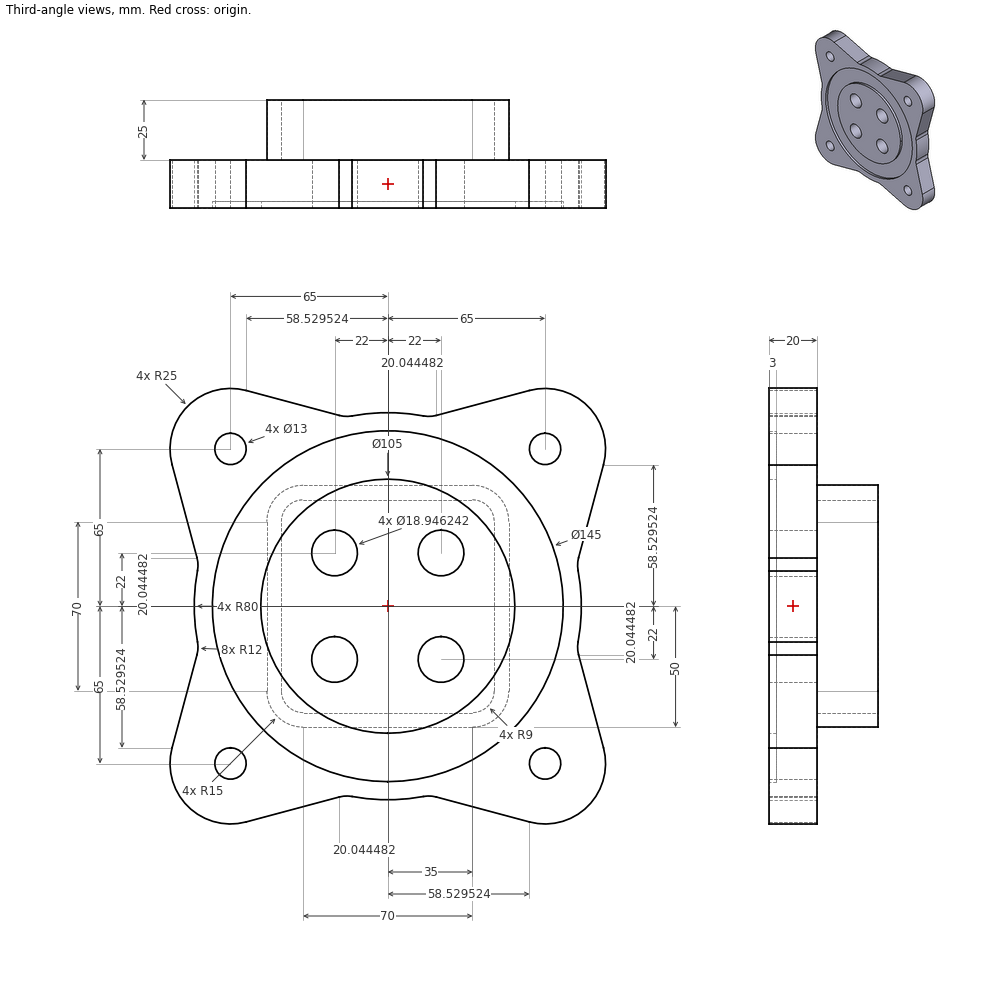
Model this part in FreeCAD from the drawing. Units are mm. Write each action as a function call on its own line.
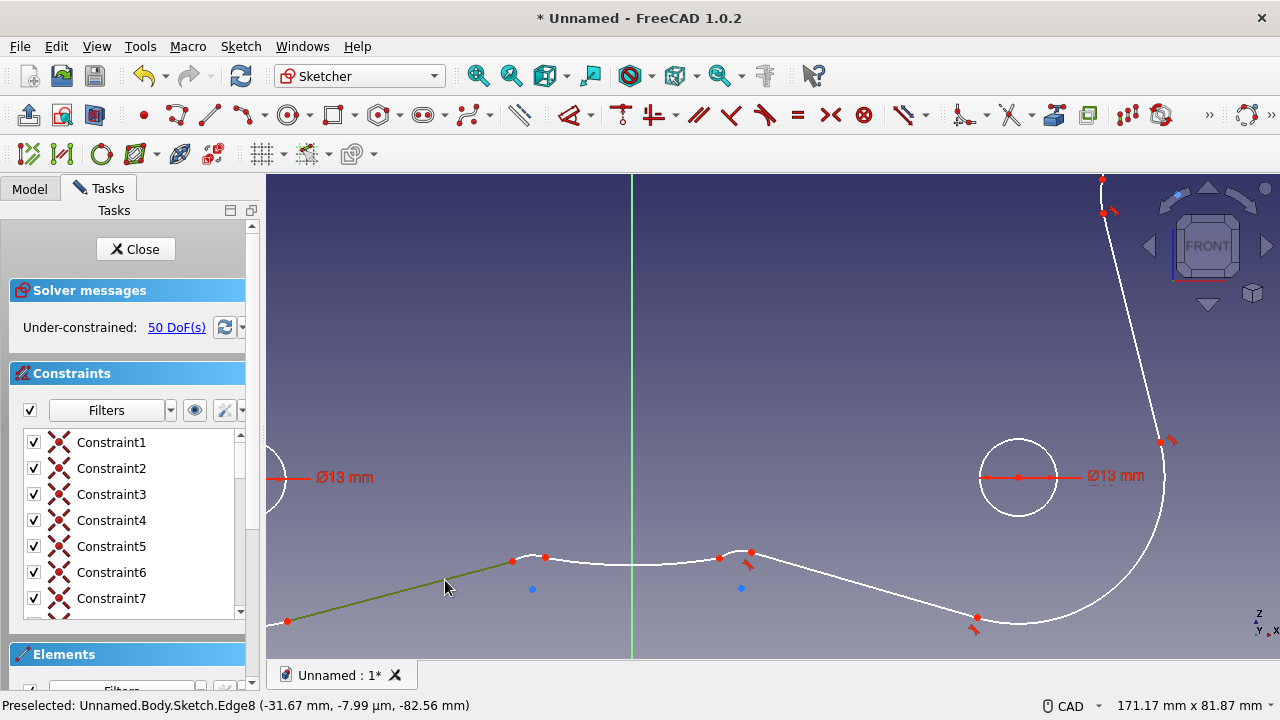
scroll(536, 555, up, 2)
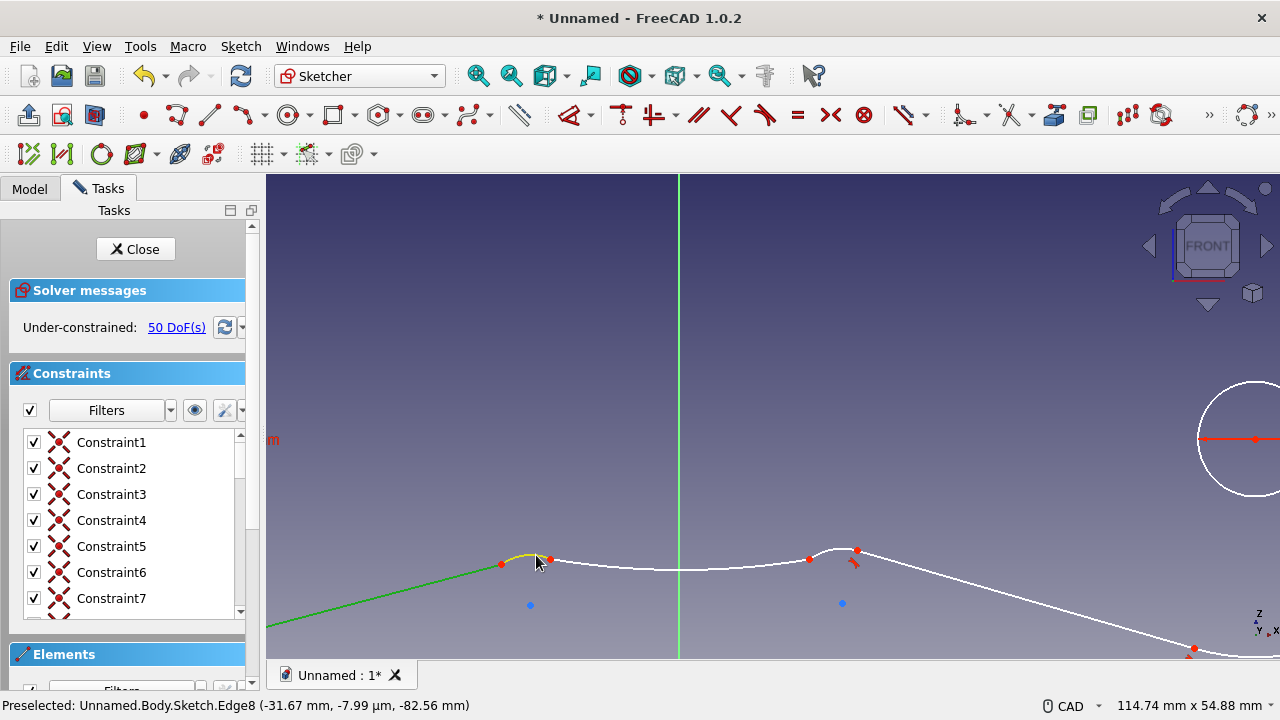
click(535, 555)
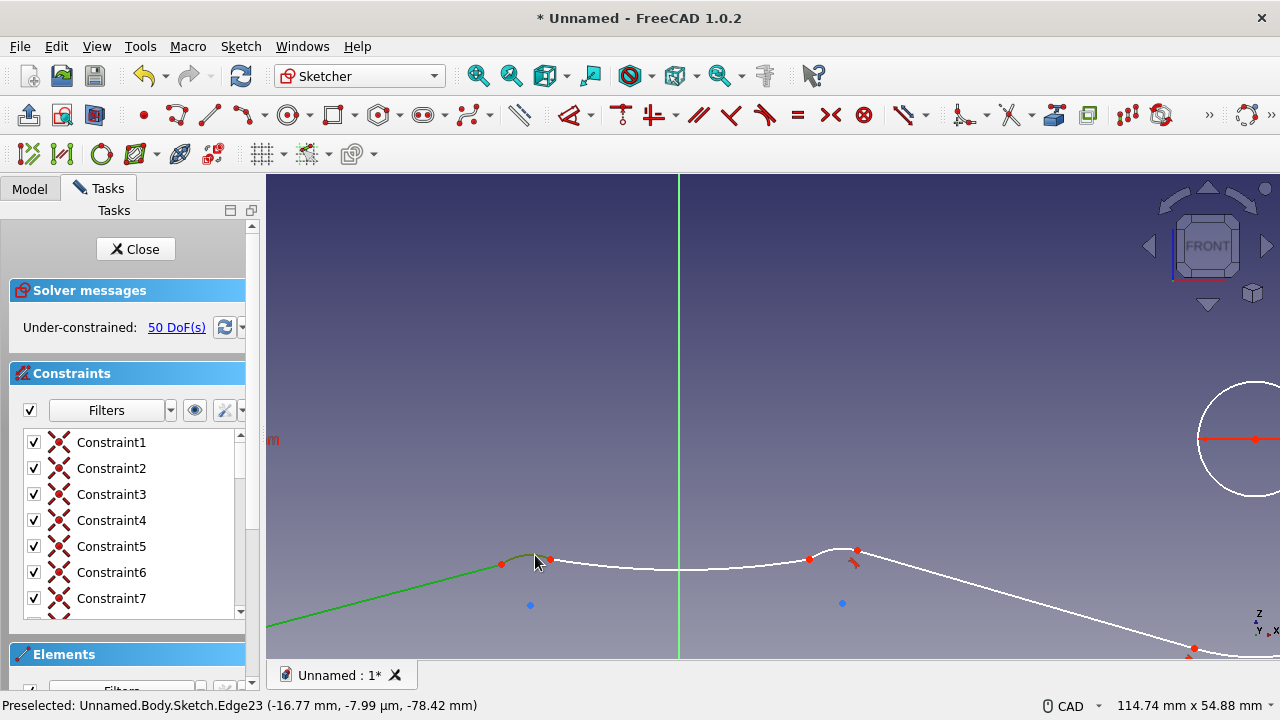
click(765, 116)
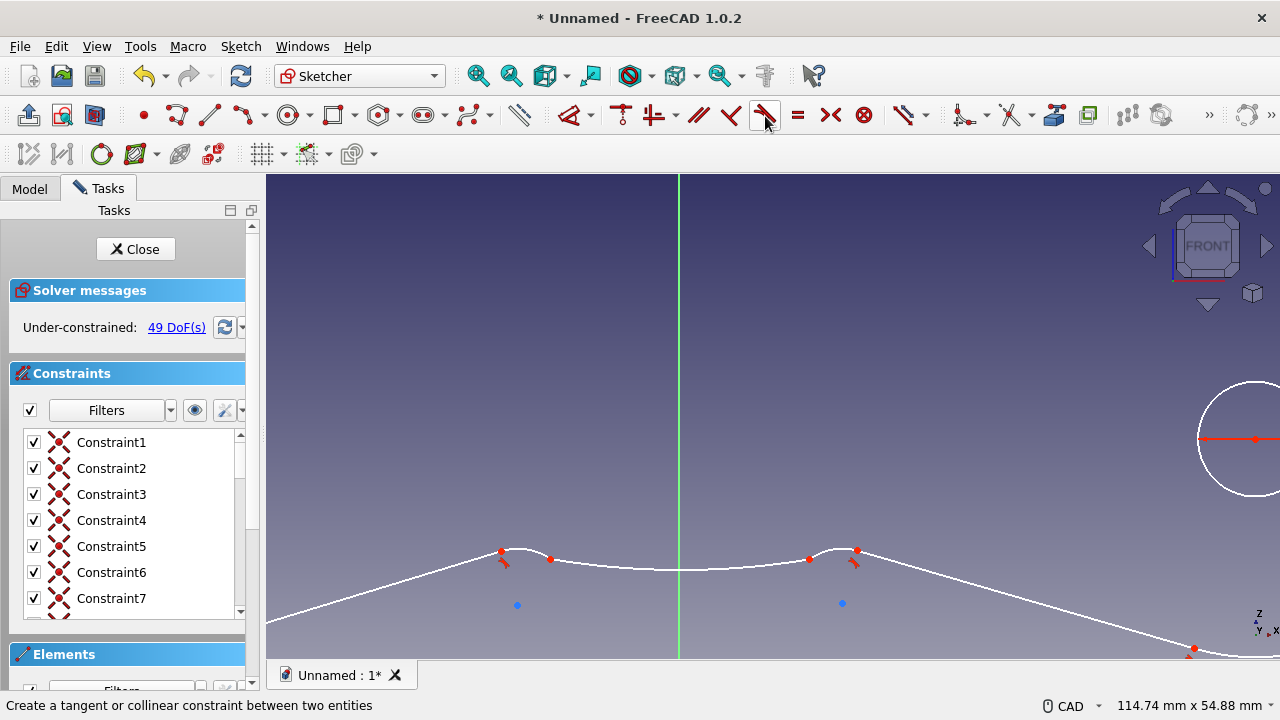
scroll(711, 557, down, 8)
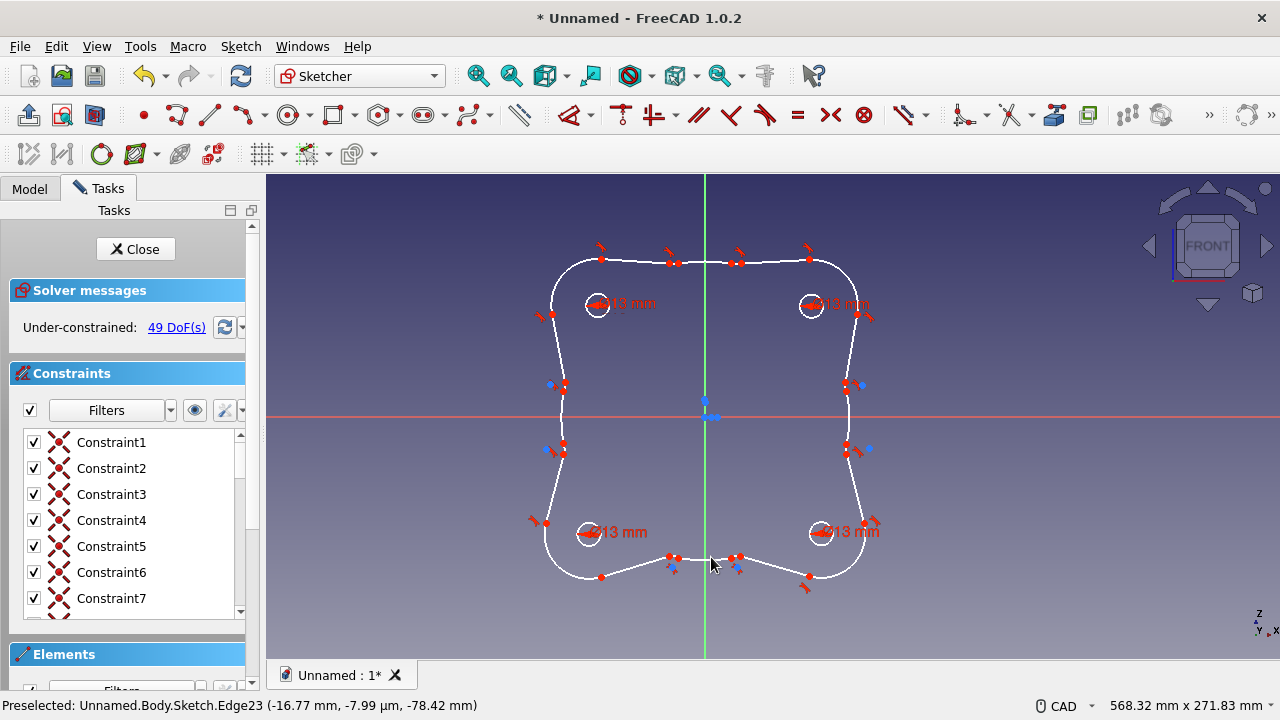
click(649, 563)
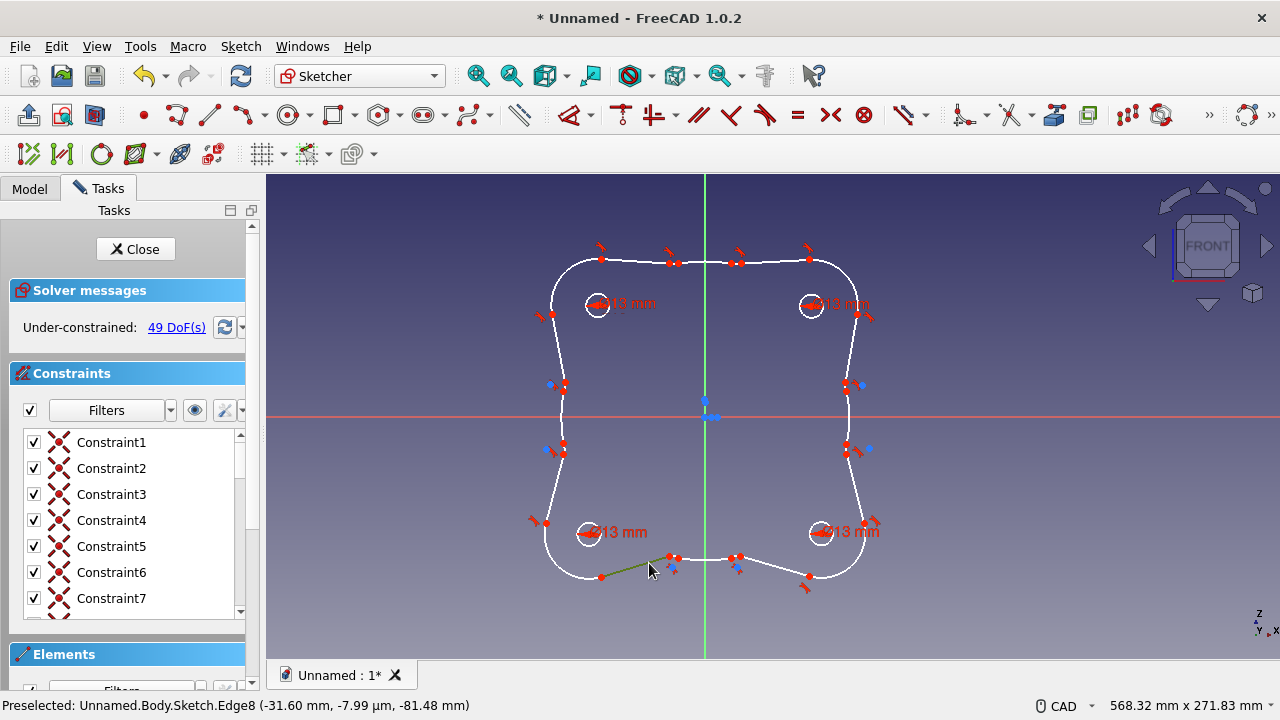
click(548, 551)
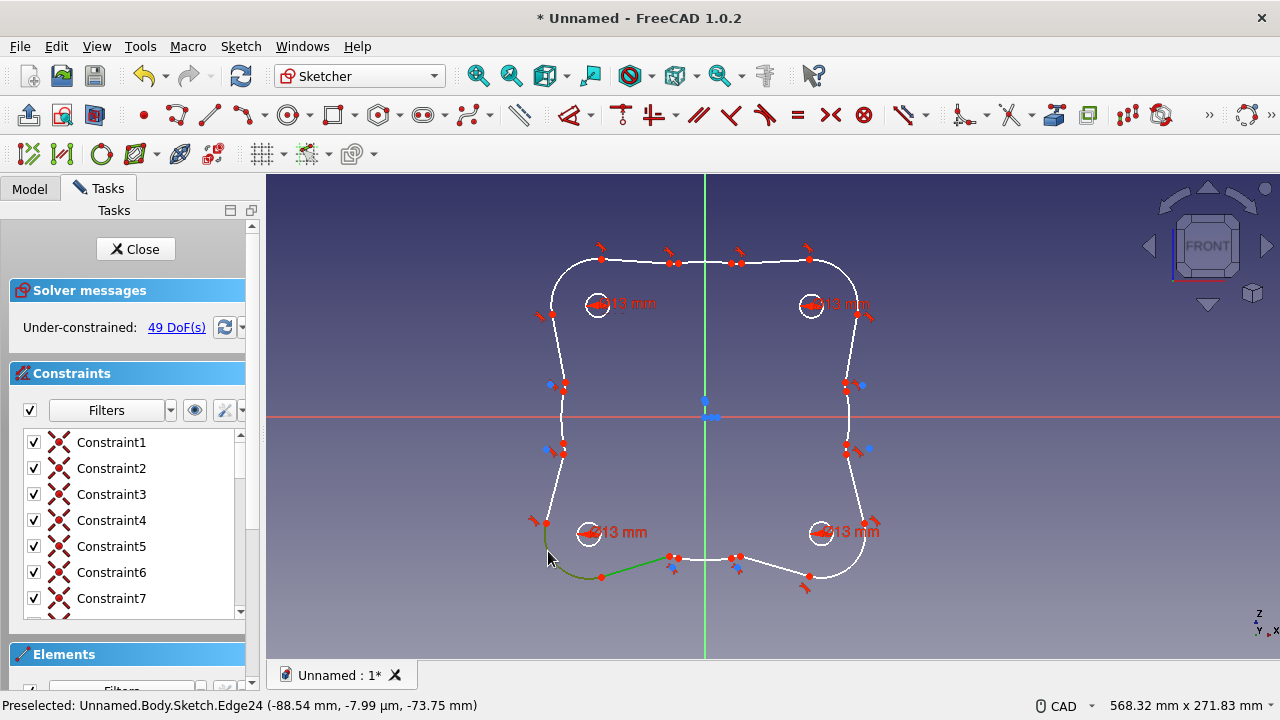
click(765, 116)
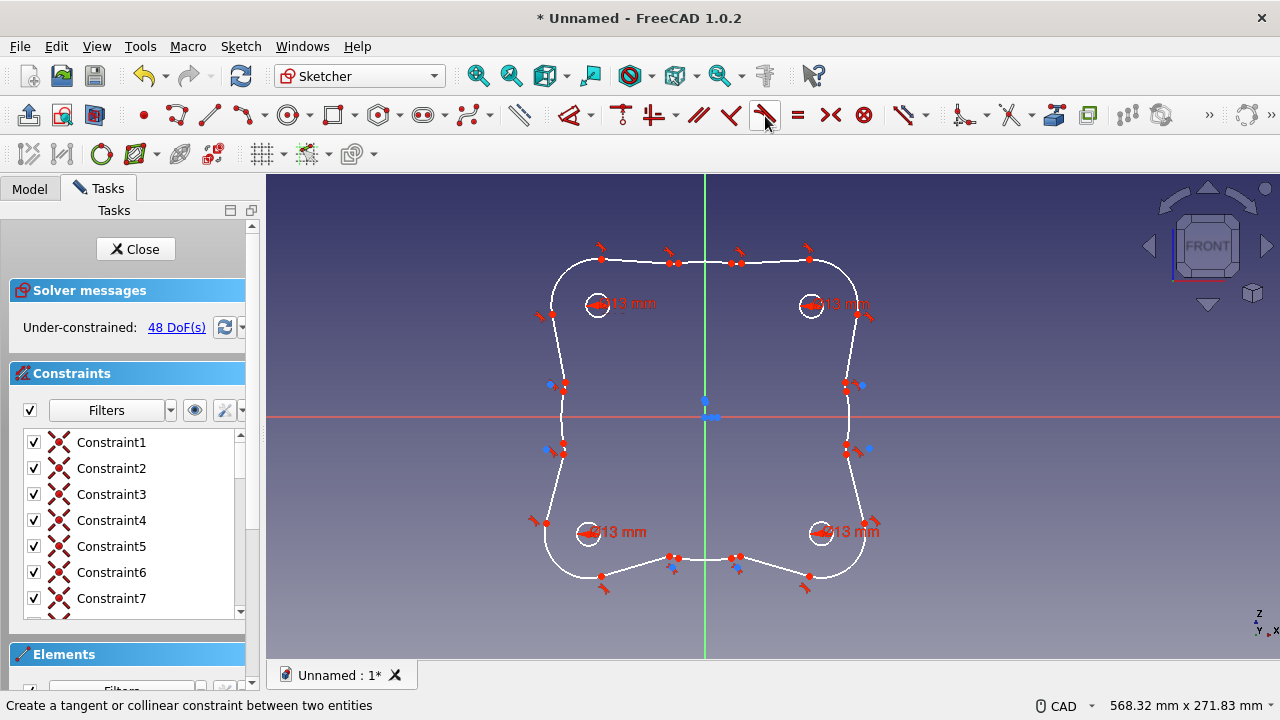
scroll(565, 449, up, 5)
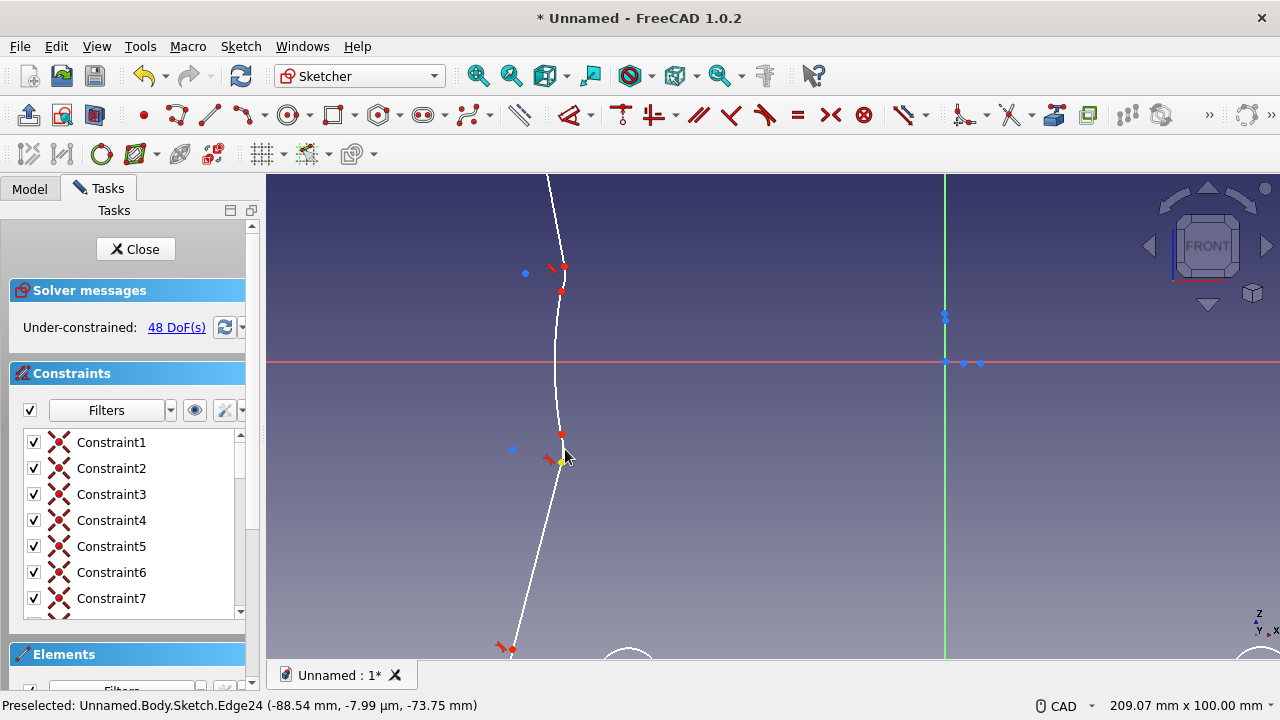
click(563, 448)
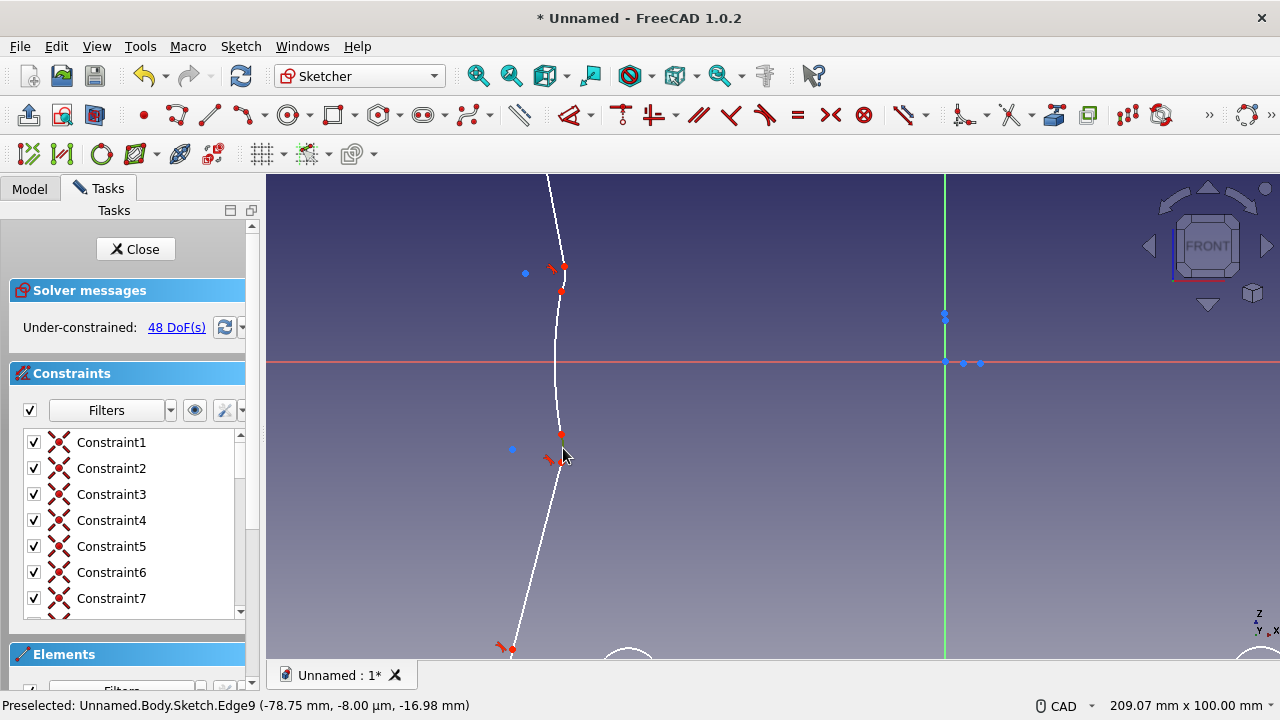
click(556, 335)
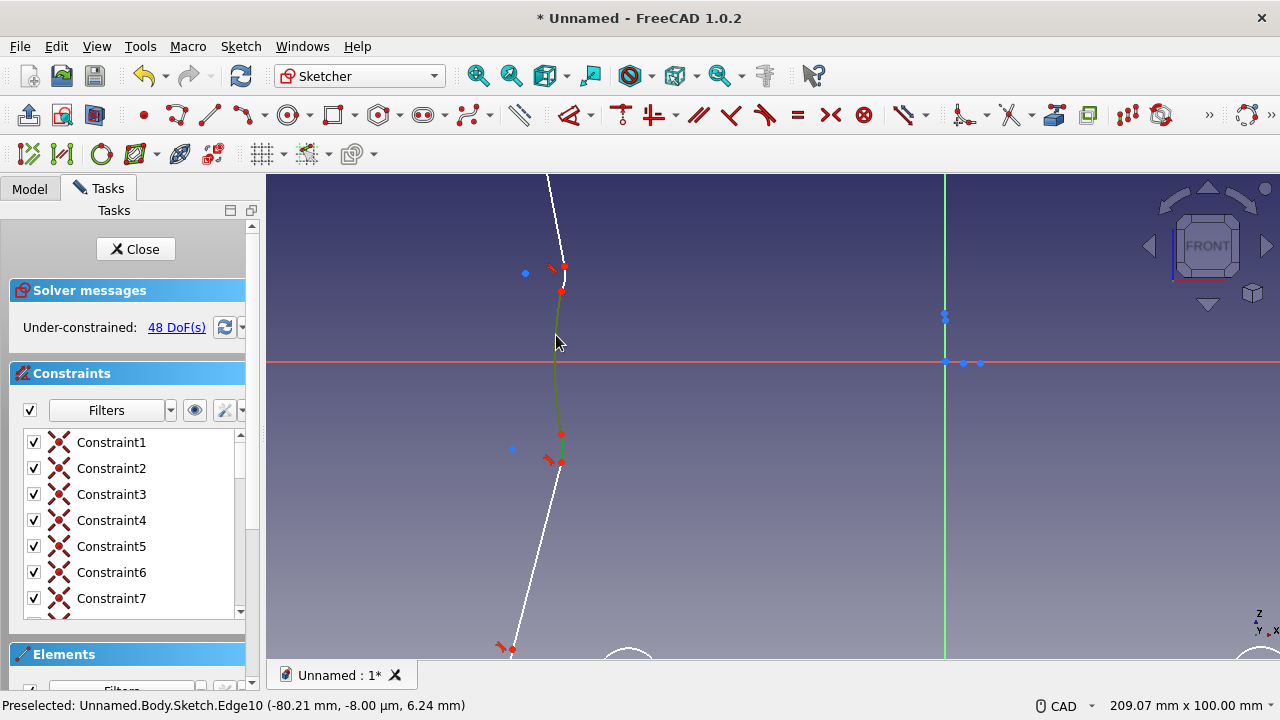
click(765, 116)